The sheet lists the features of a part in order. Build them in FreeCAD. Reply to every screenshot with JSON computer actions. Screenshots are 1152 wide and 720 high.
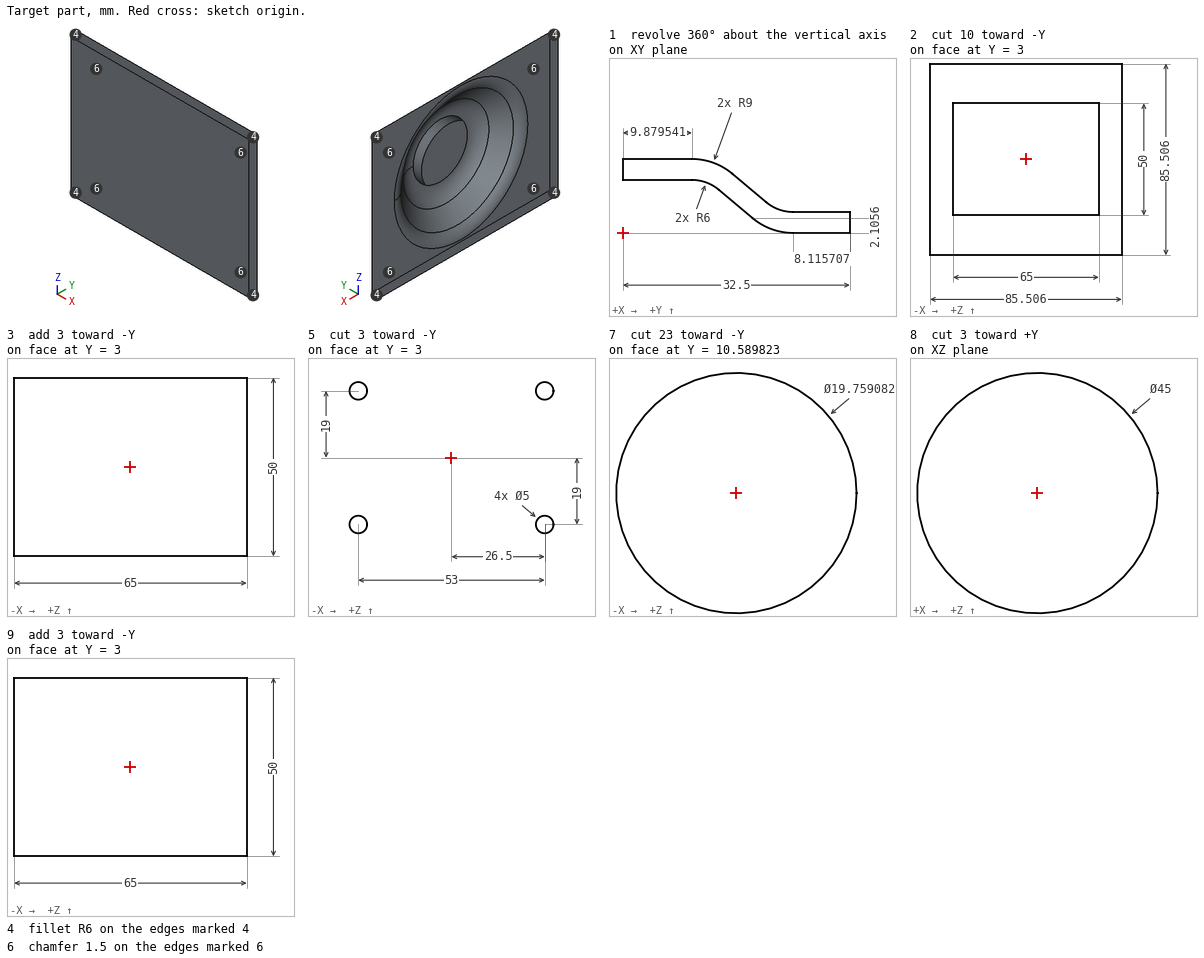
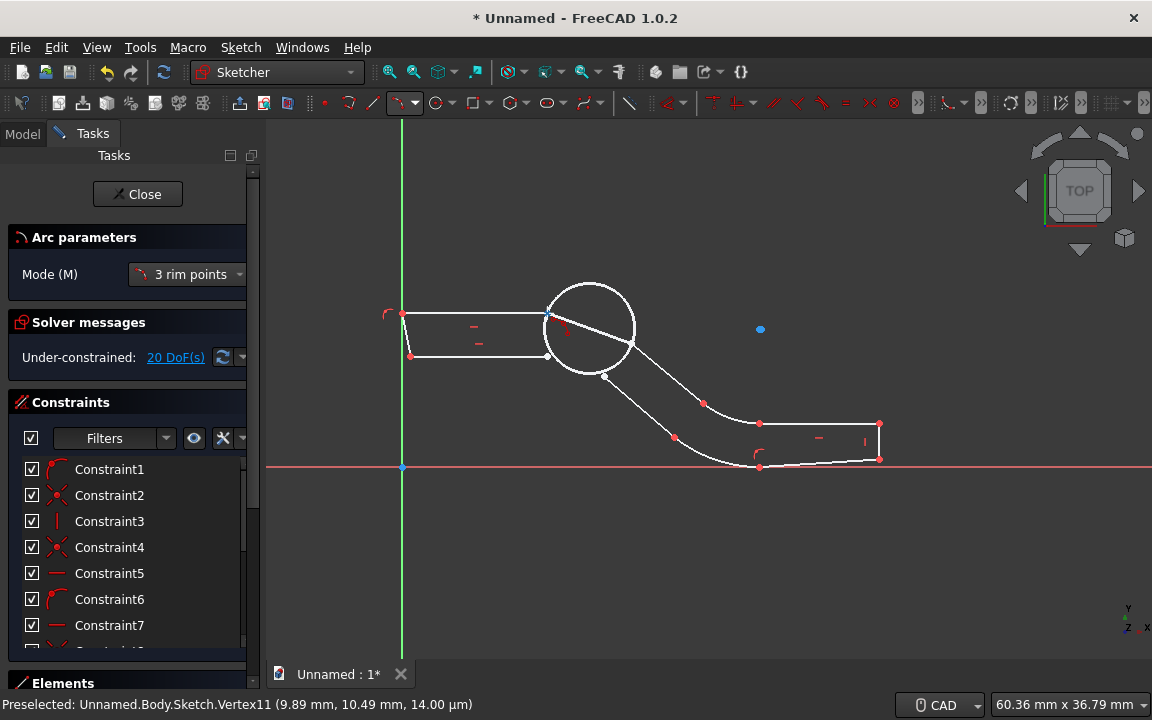
{"action": "scroll", "coordinate": [592, 320], "scroll_direction": "up", "scroll_amount": 4}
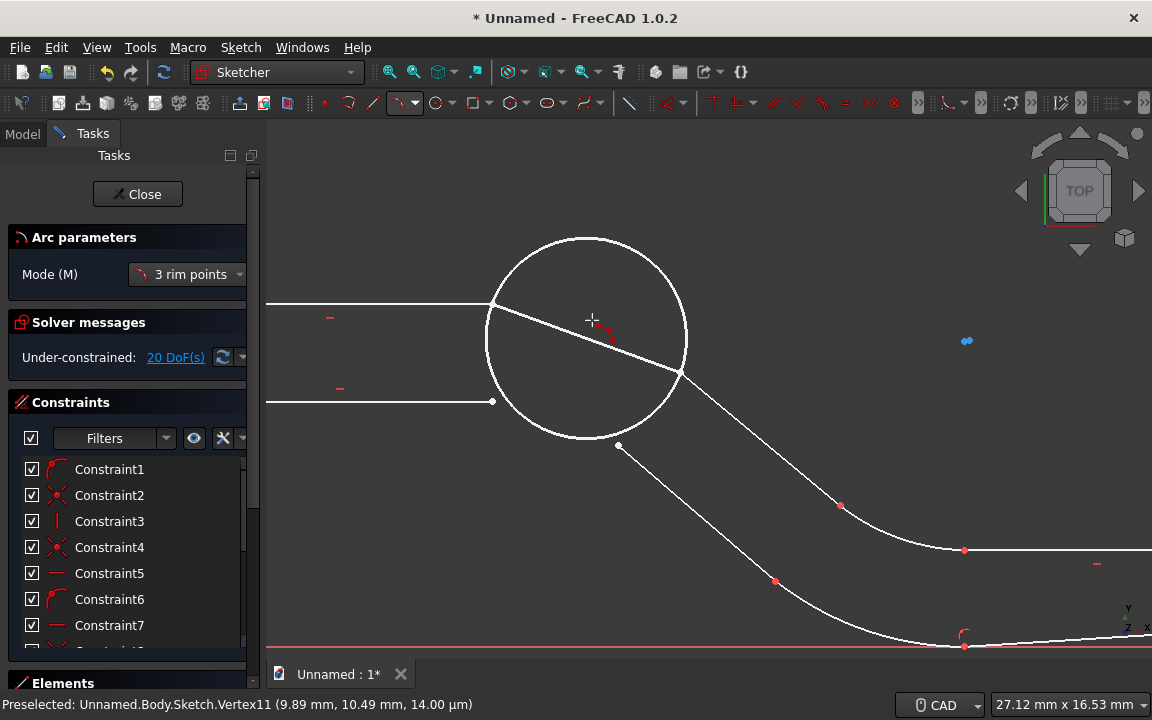
{"action": "left_click", "coordinate": [592, 319]}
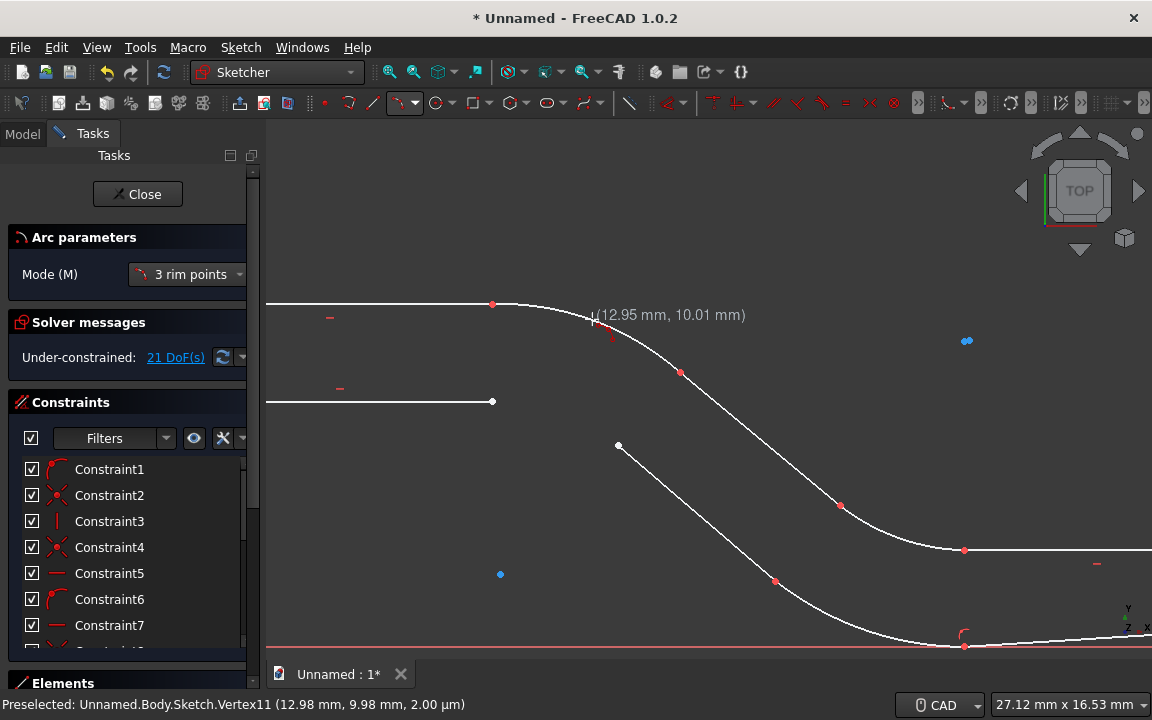
{"action": "left_click", "coordinate": [492, 402]}
{"action": "left_click", "coordinate": [618, 446]}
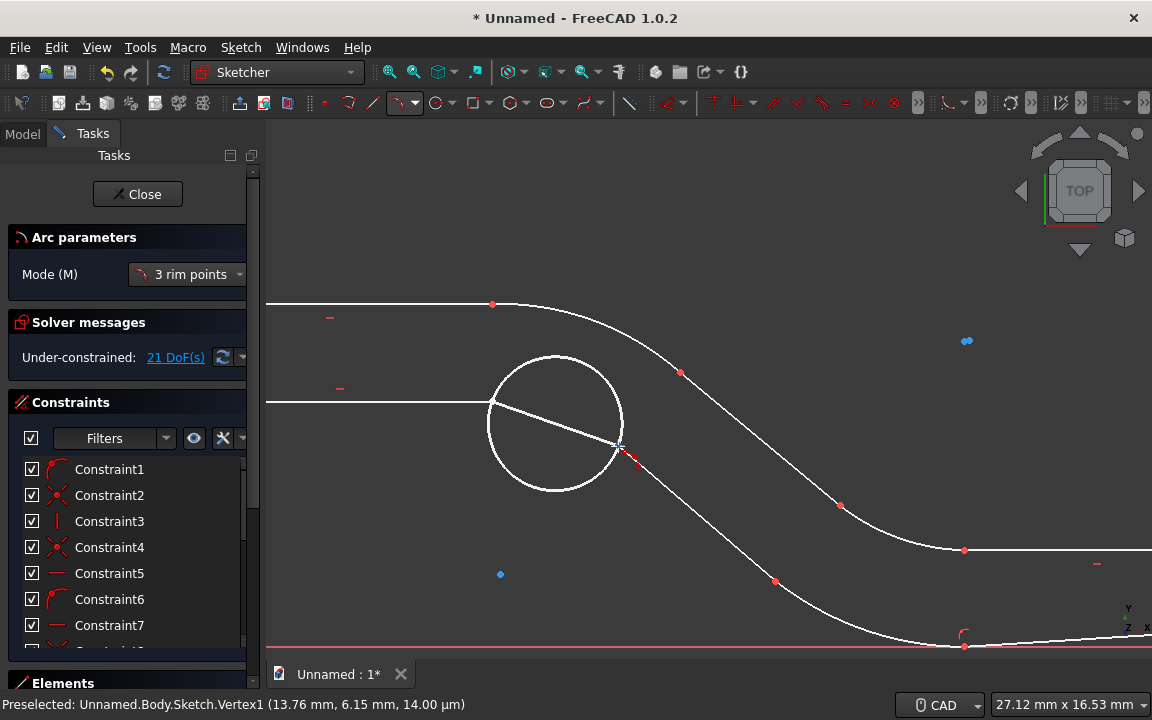
{"action": "scroll", "coordinate": [559, 411], "scroll_direction": "up", "scroll_amount": 2}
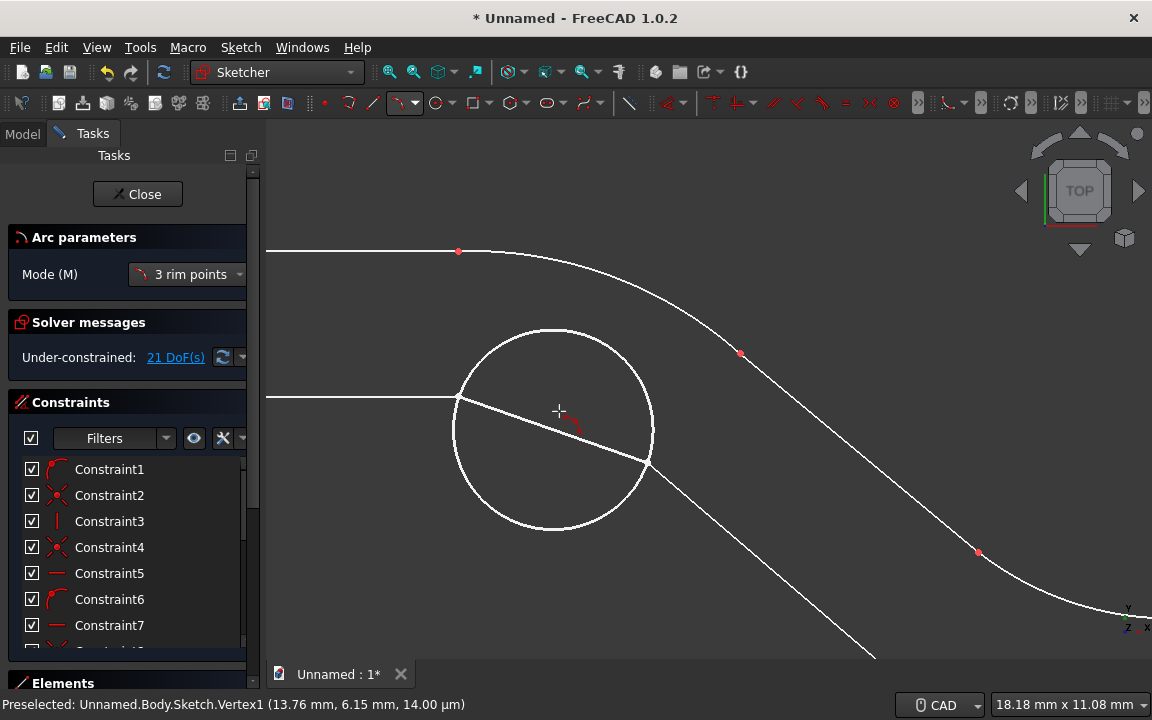
{"action": "left_click", "coordinate": [558, 410]}
{"action": "key", "text": "Escape"}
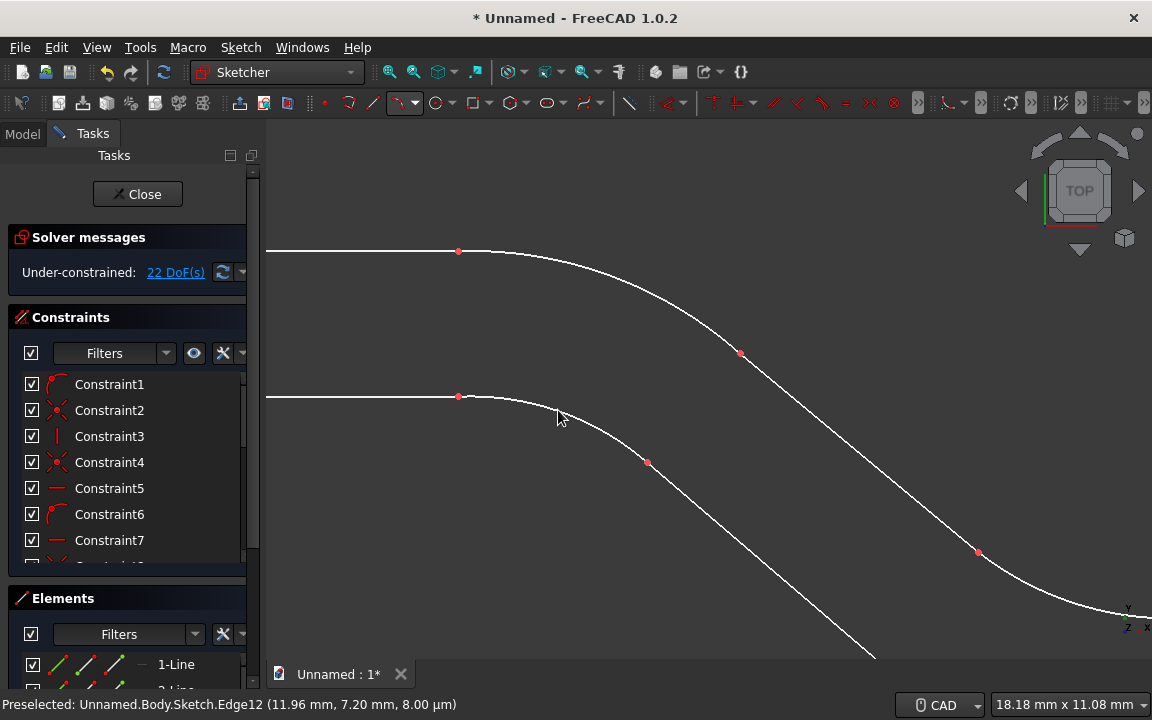
{"action": "left_click", "coordinate": [718, 523]}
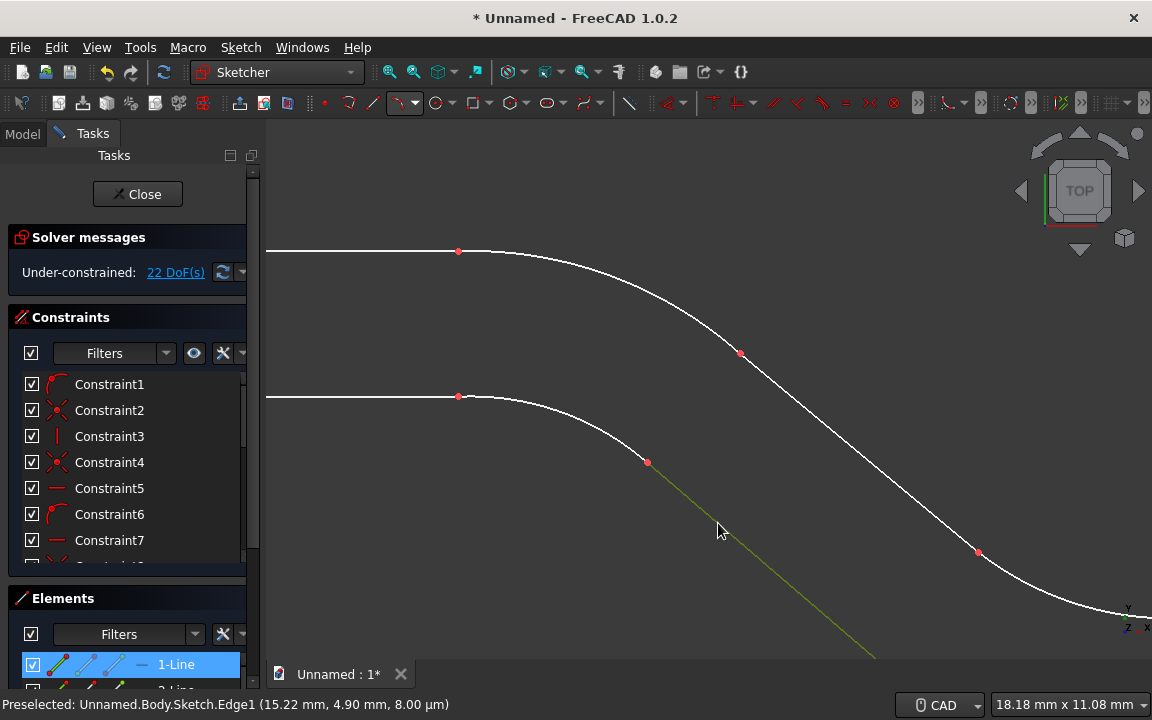
{"action": "scroll", "coordinate": [585, 339], "scroll_direction": "down", "scroll_amount": 6}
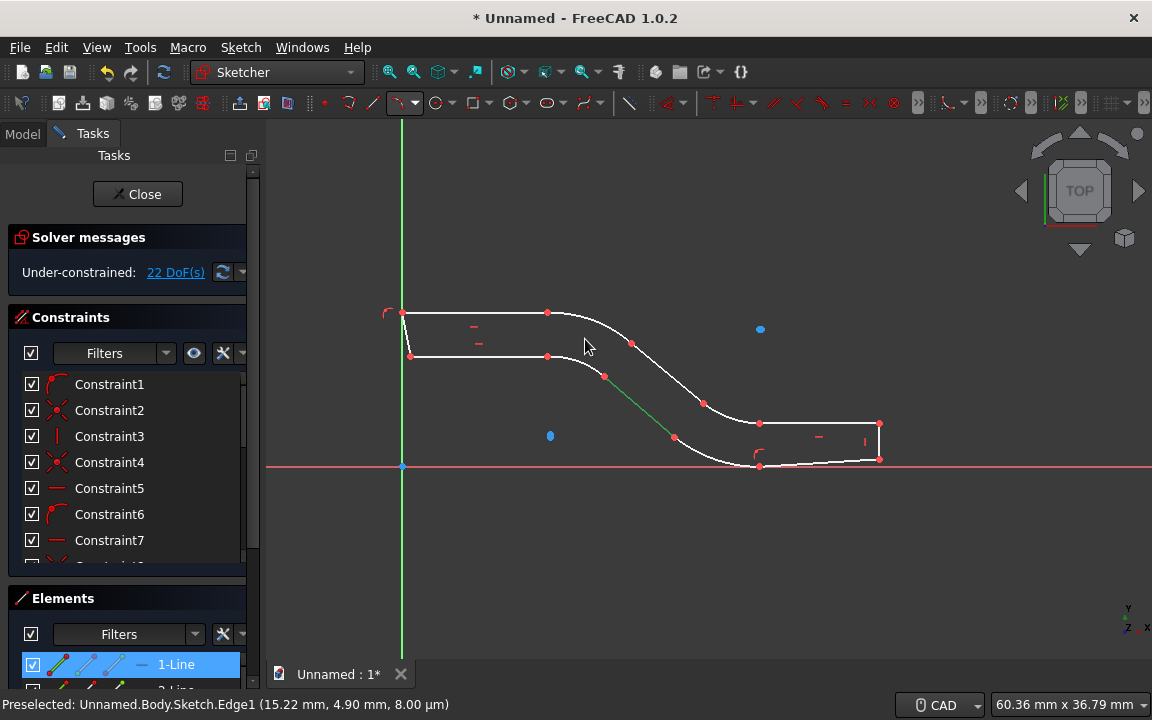
{"action": "left_click", "coordinate": [698, 452]}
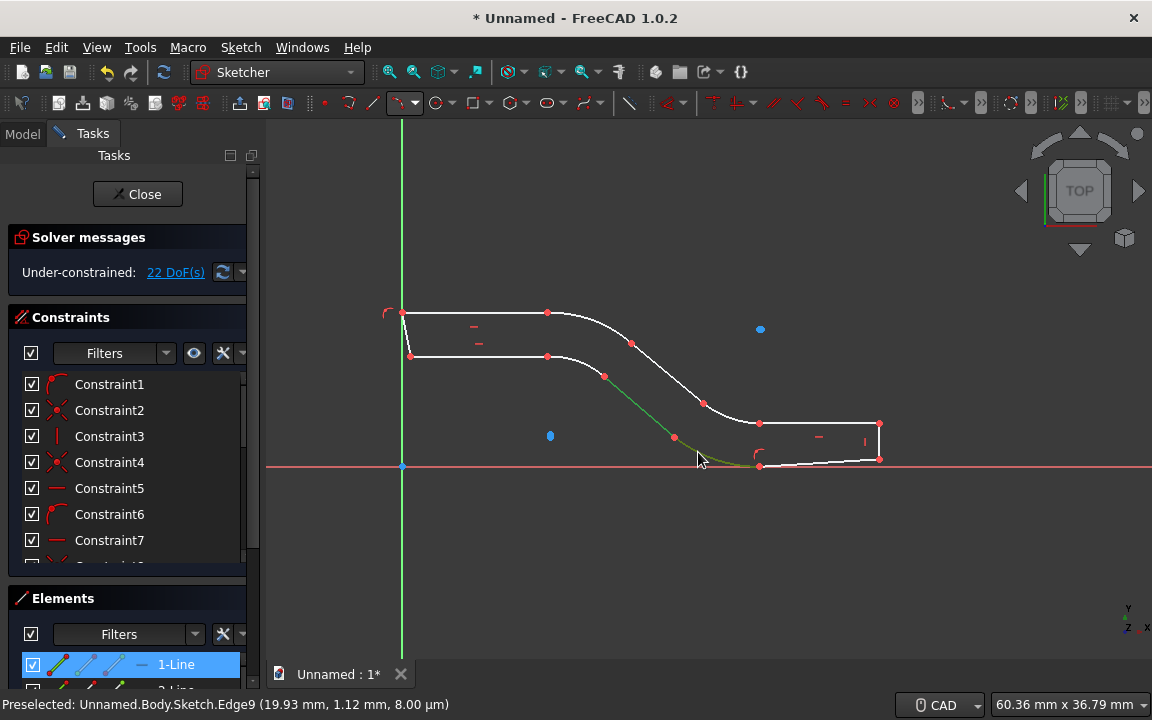
{"action": "left_click", "coordinate": [822, 104]}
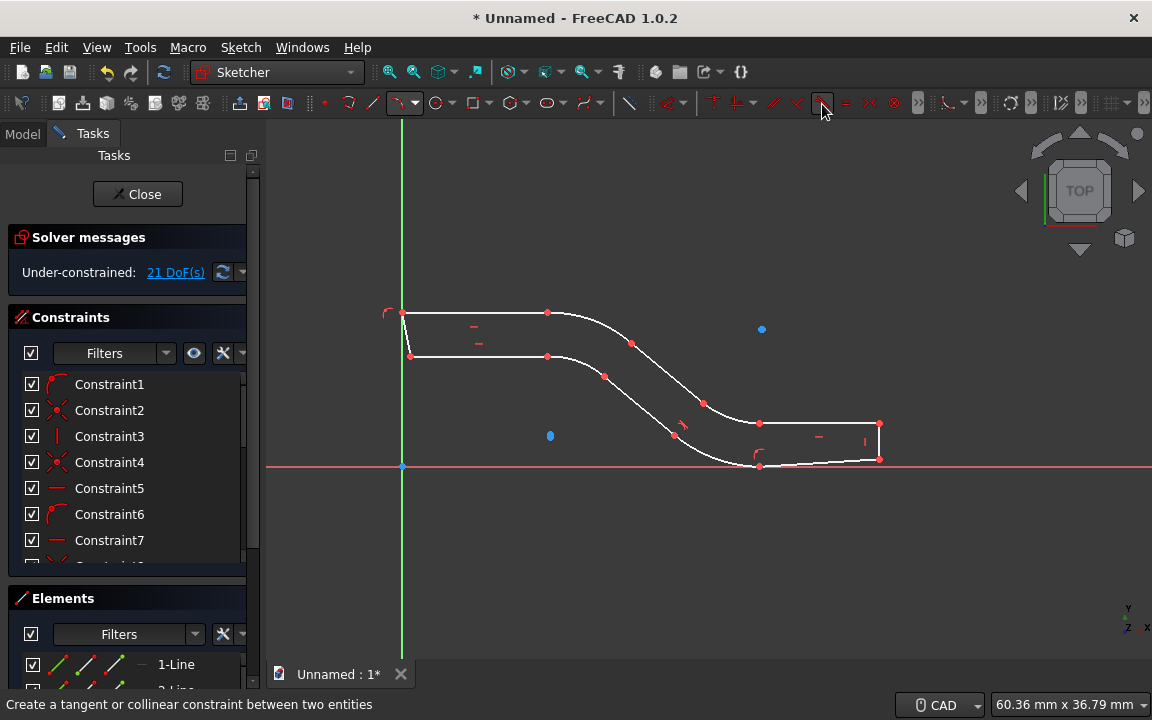
{"action": "left_click", "coordinate": [625, 394]}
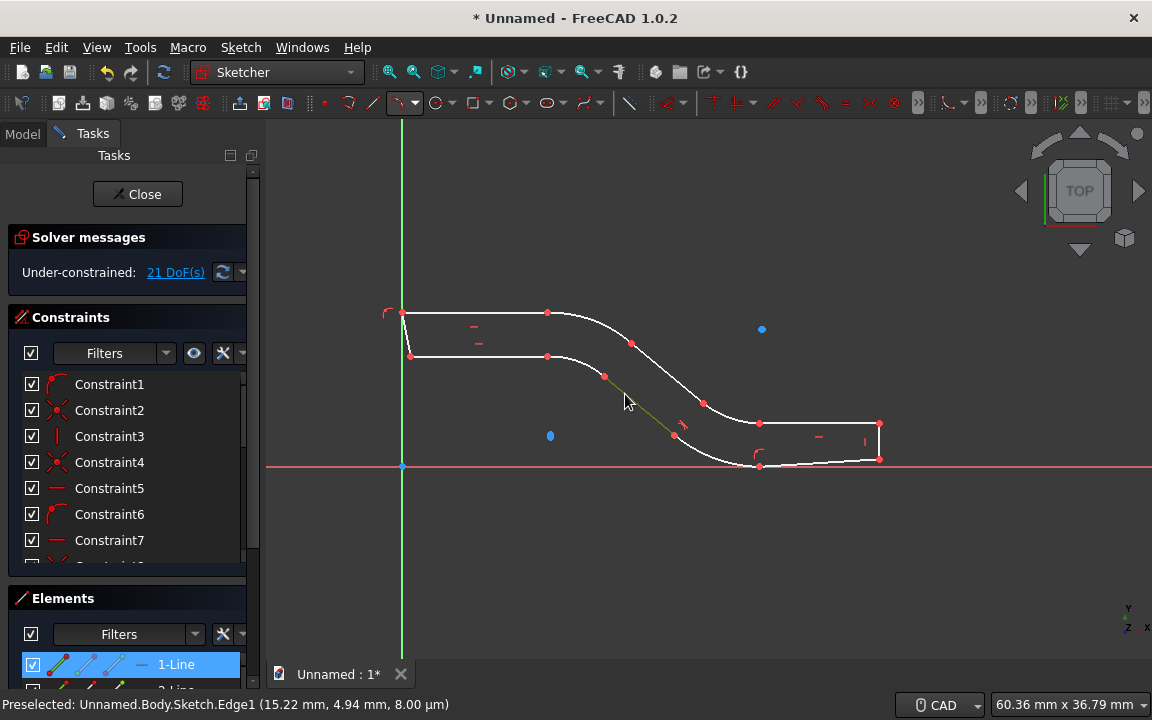
{"action": "left_click", "coordinate": [589, 366]}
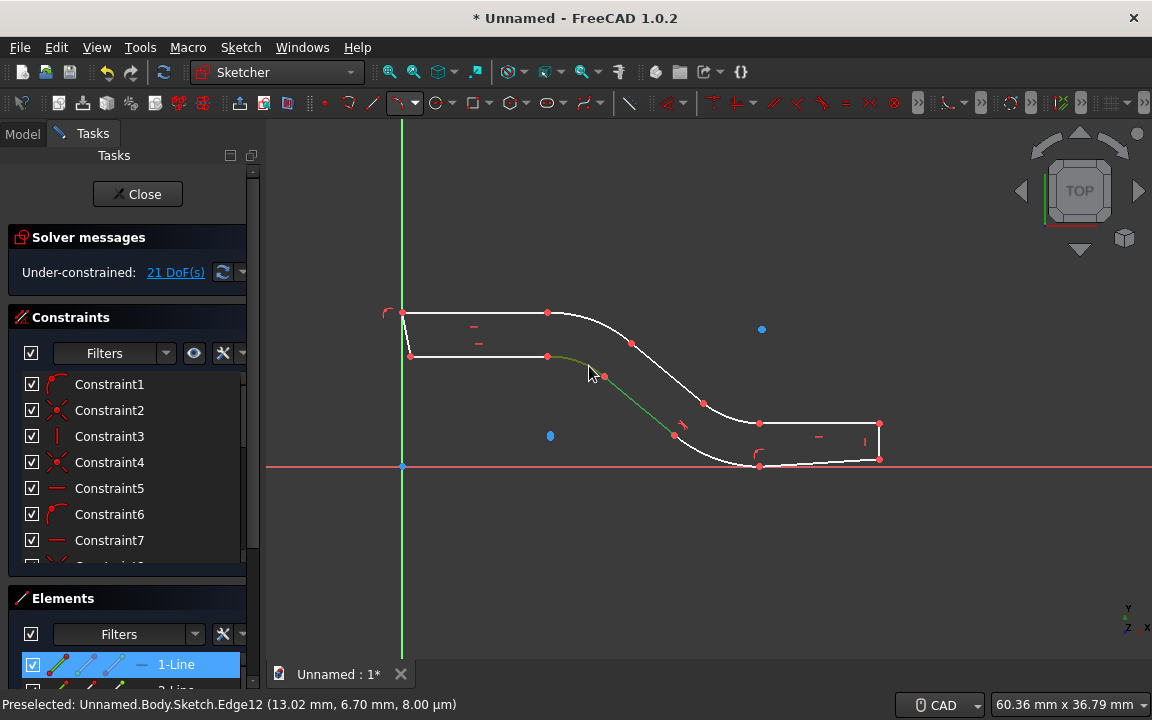
{"action": "left_click", "coordinate": [822, 104]}